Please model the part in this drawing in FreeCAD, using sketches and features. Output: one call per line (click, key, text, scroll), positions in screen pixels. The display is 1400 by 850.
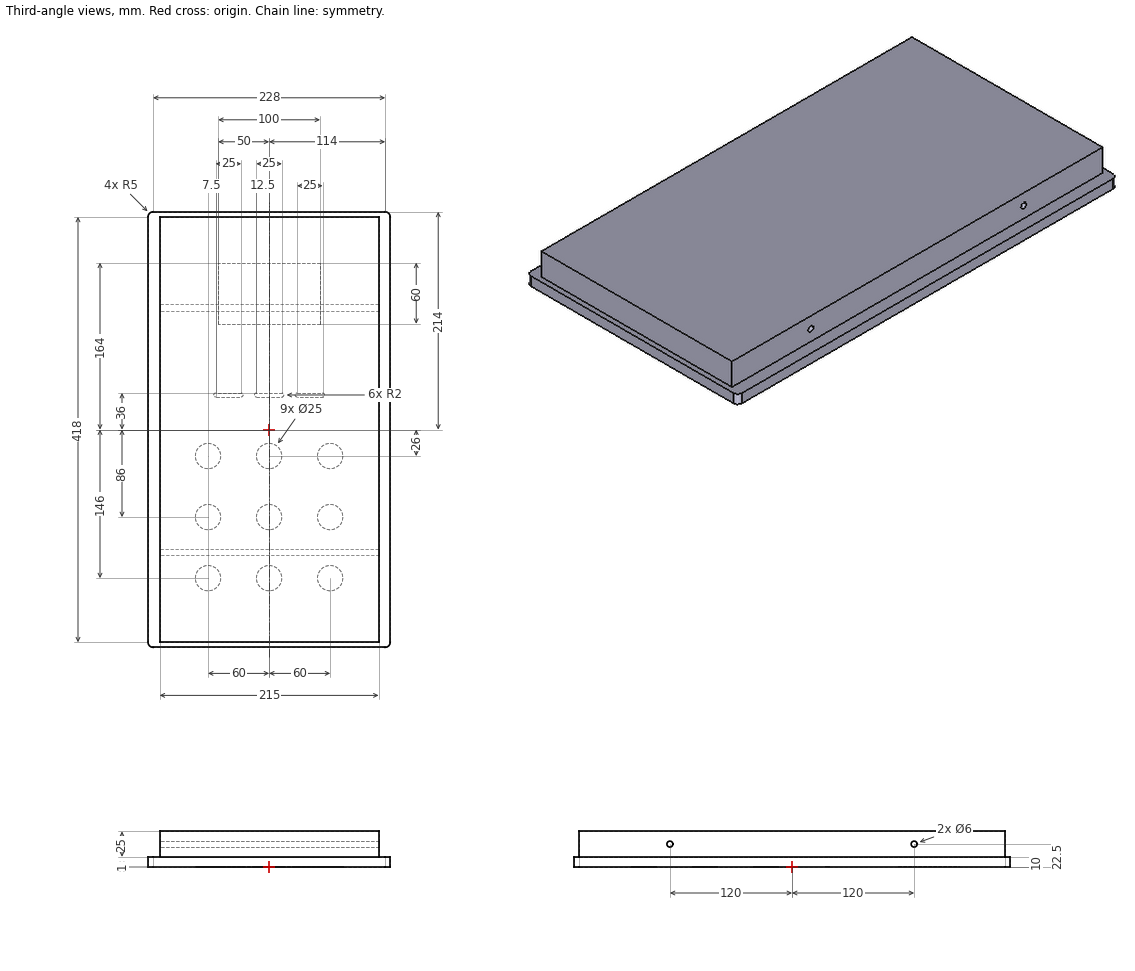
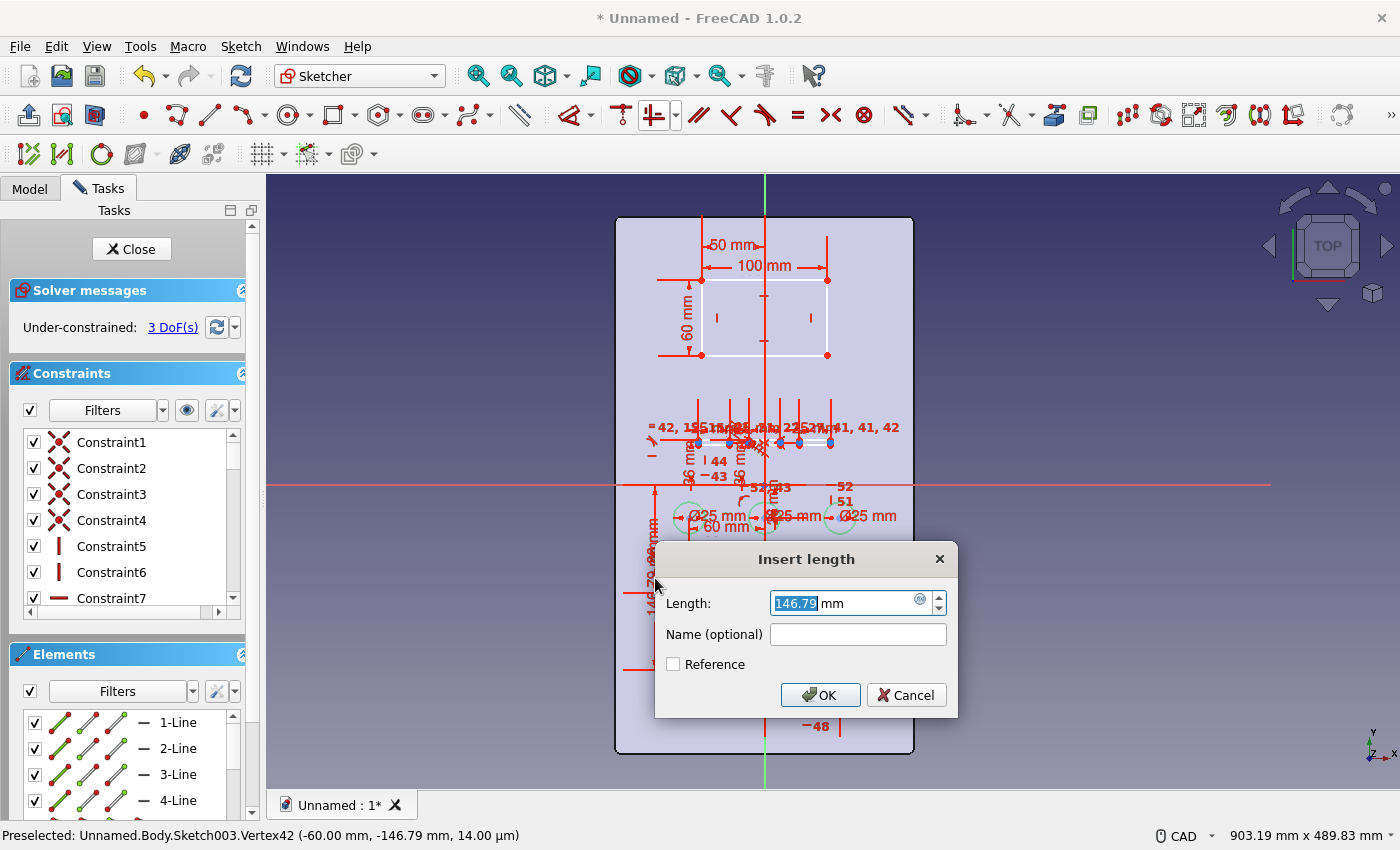
text(146)
key(Return)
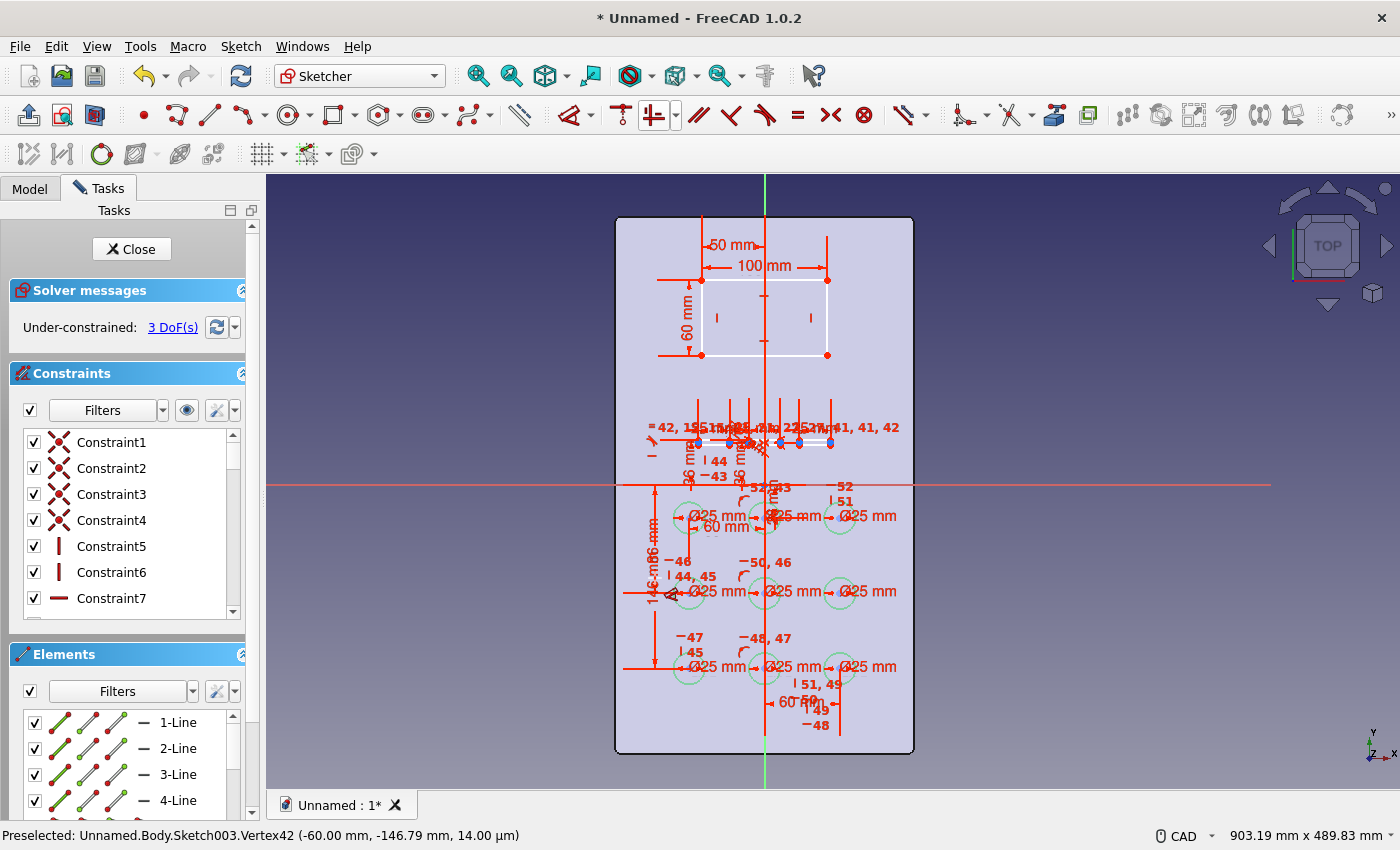
click(702, 280)
click(668, 383)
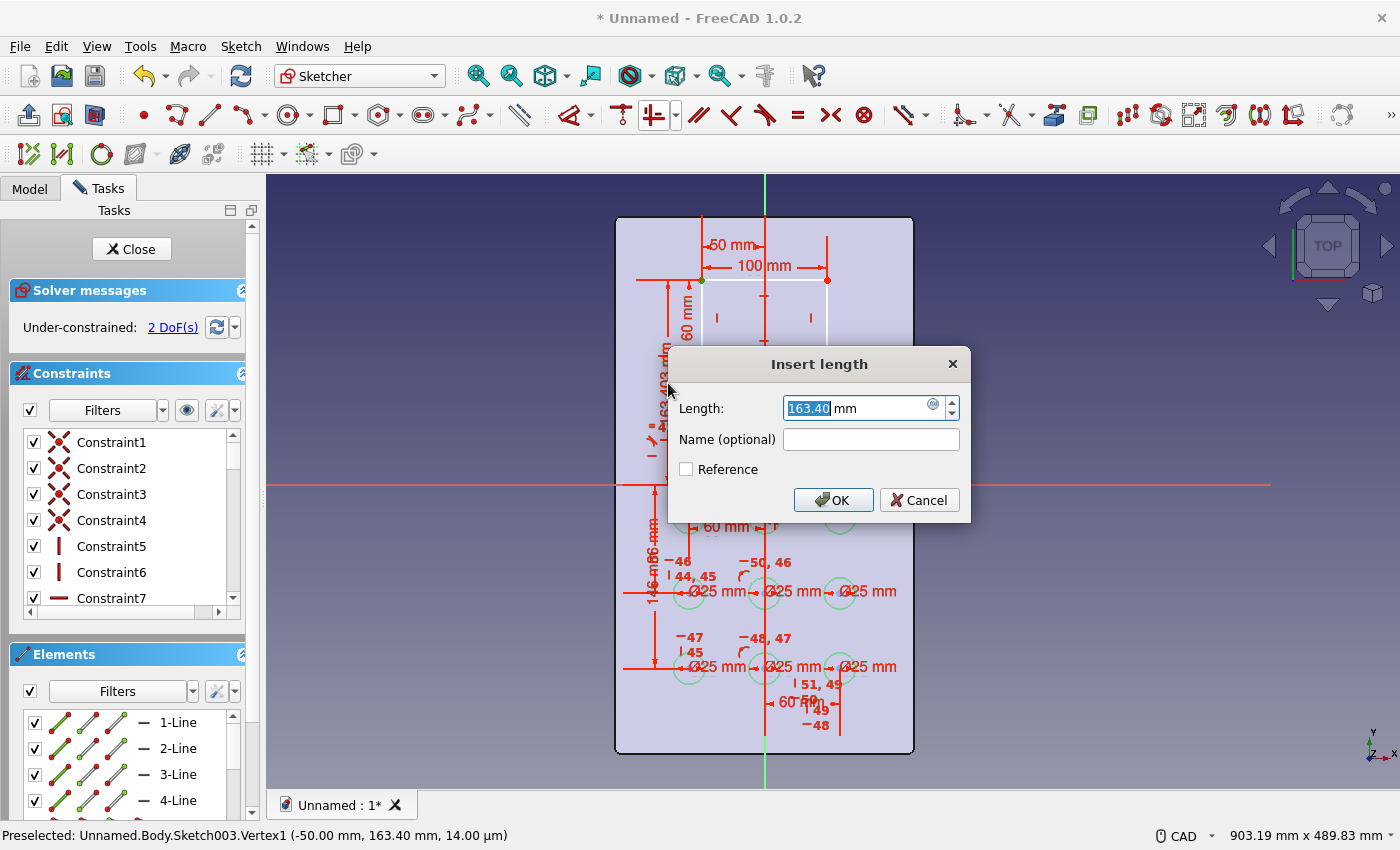
text(164)
key(Return)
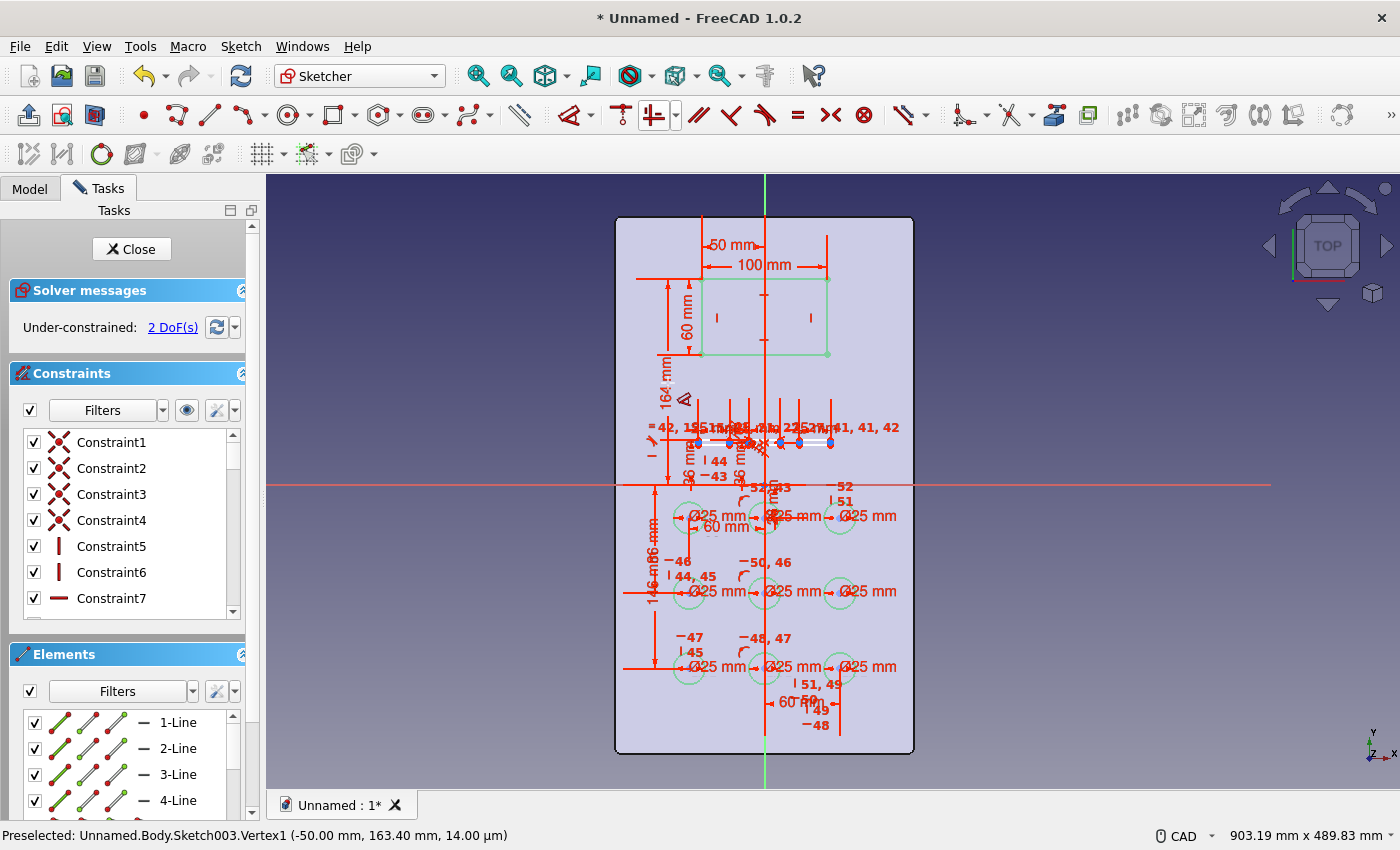
scroll(698, 445, up, 8)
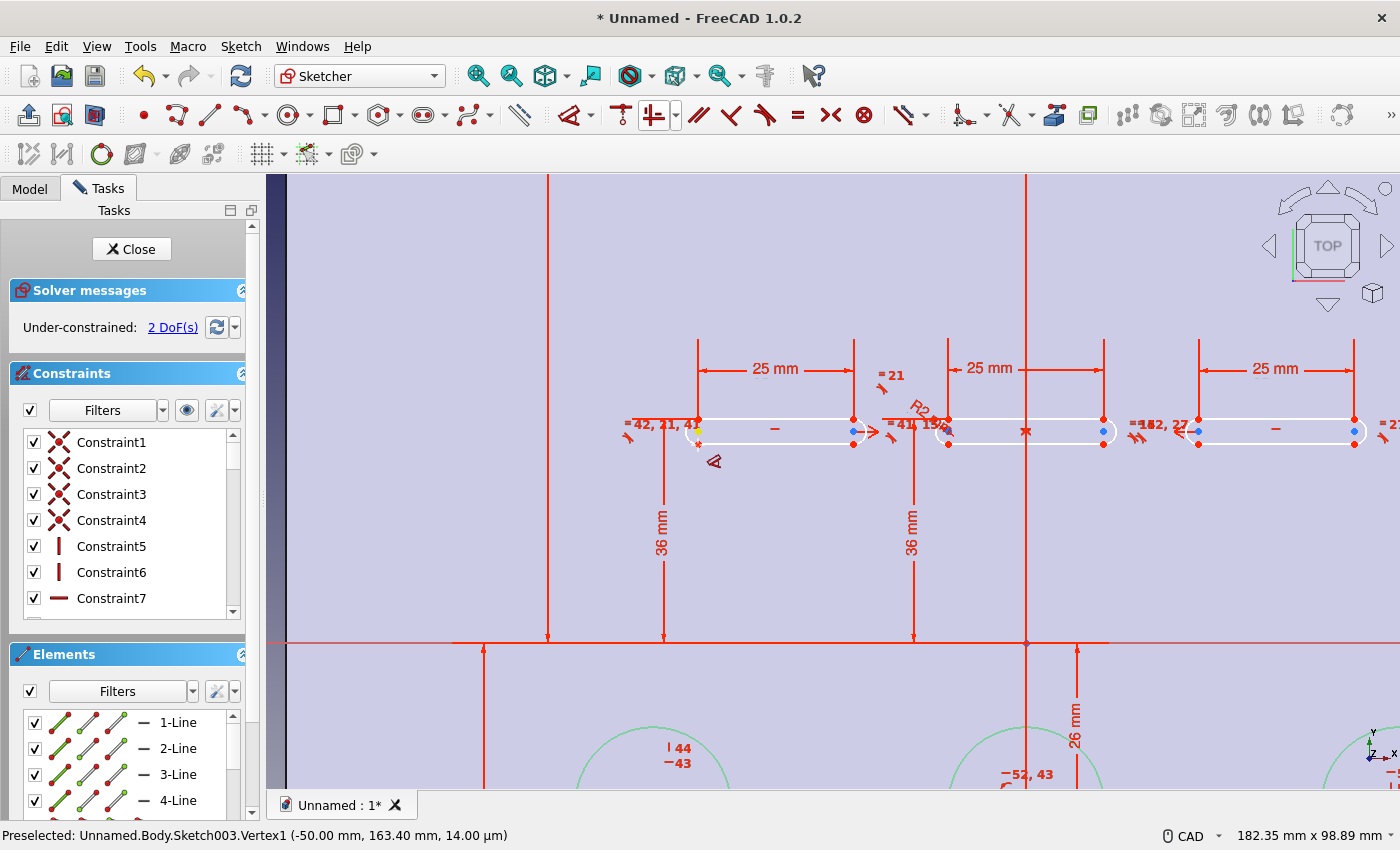
click(698, 444)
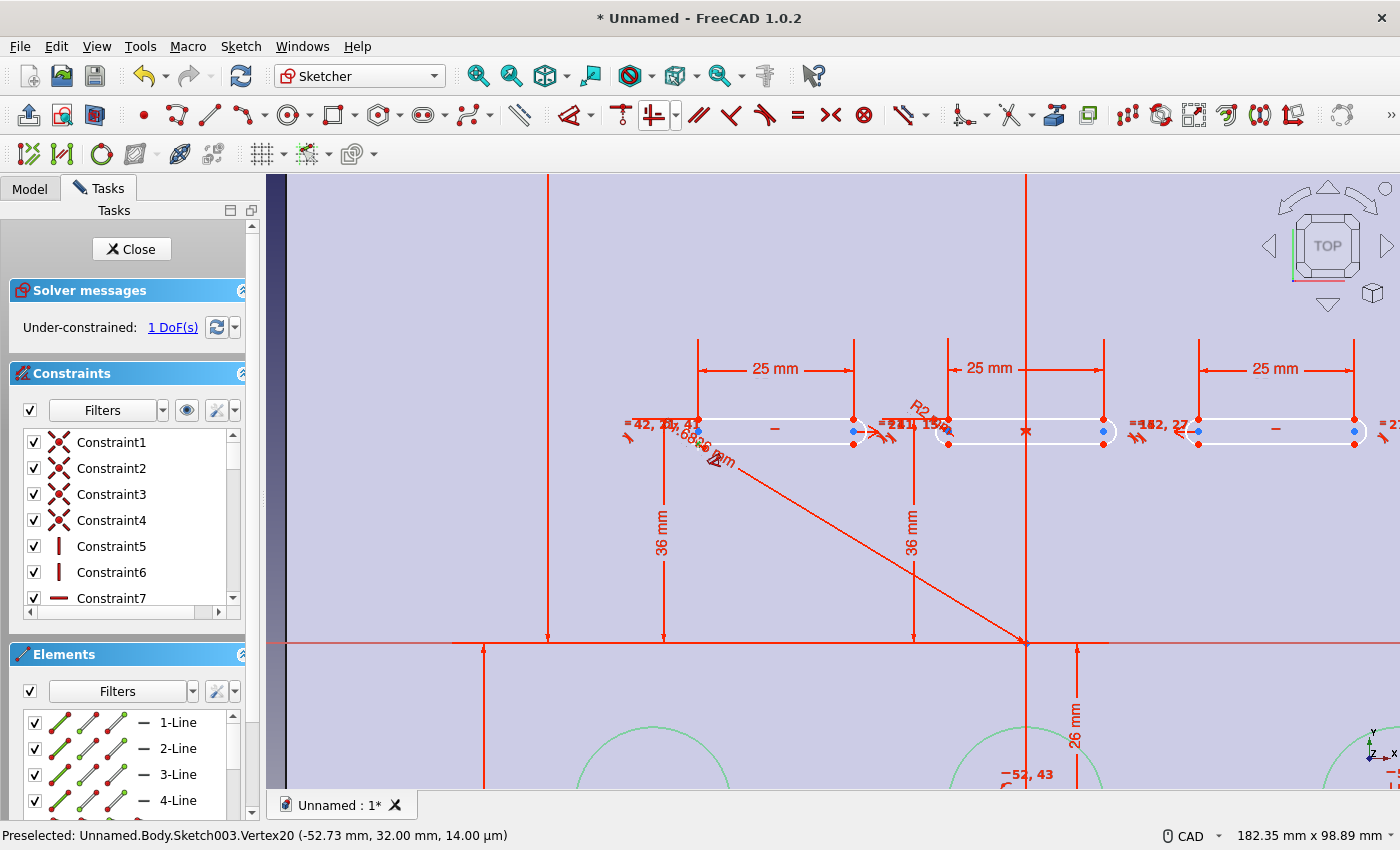
scroll(698, 445, down, 8)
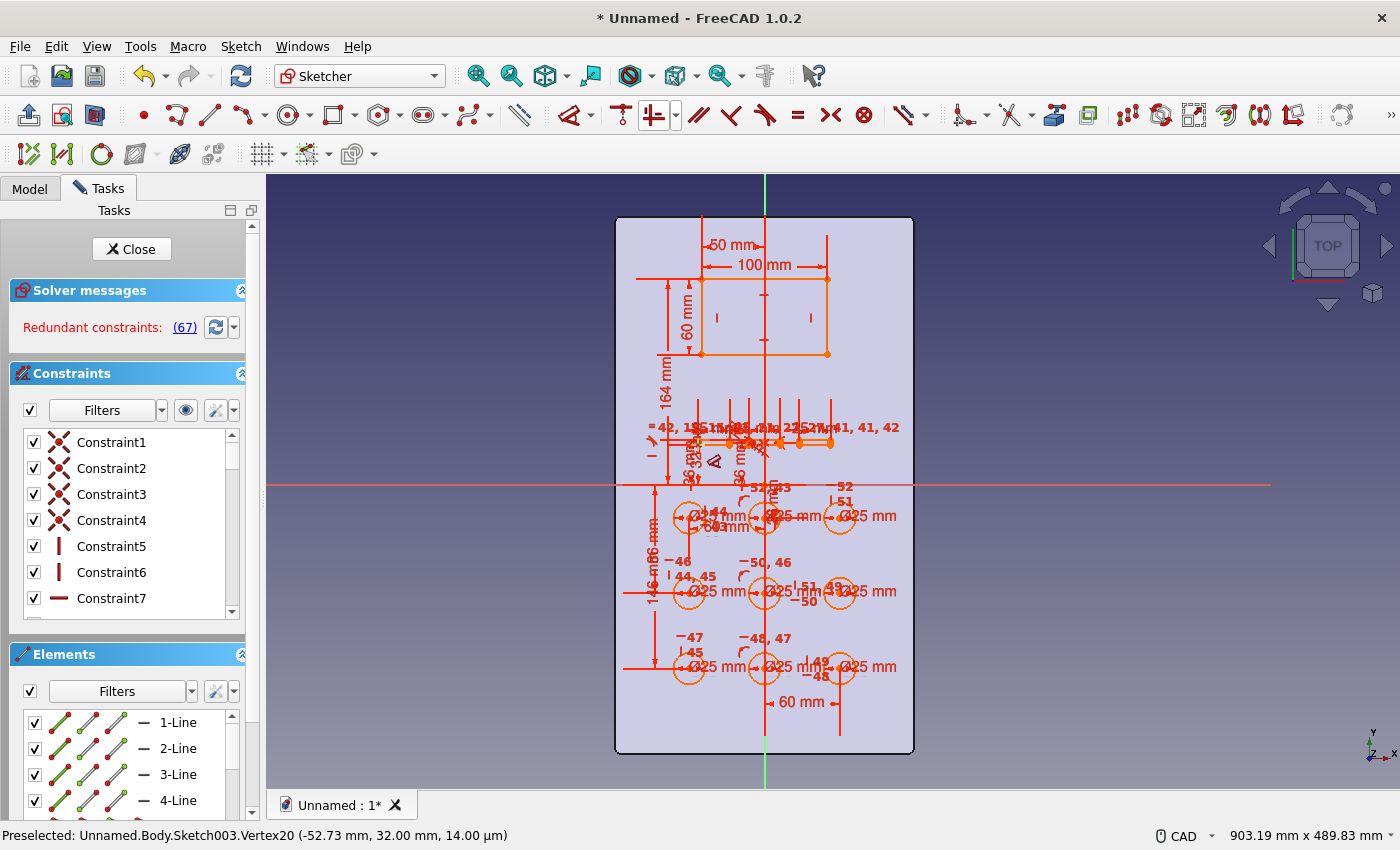
scroll(689, 518, up, 8)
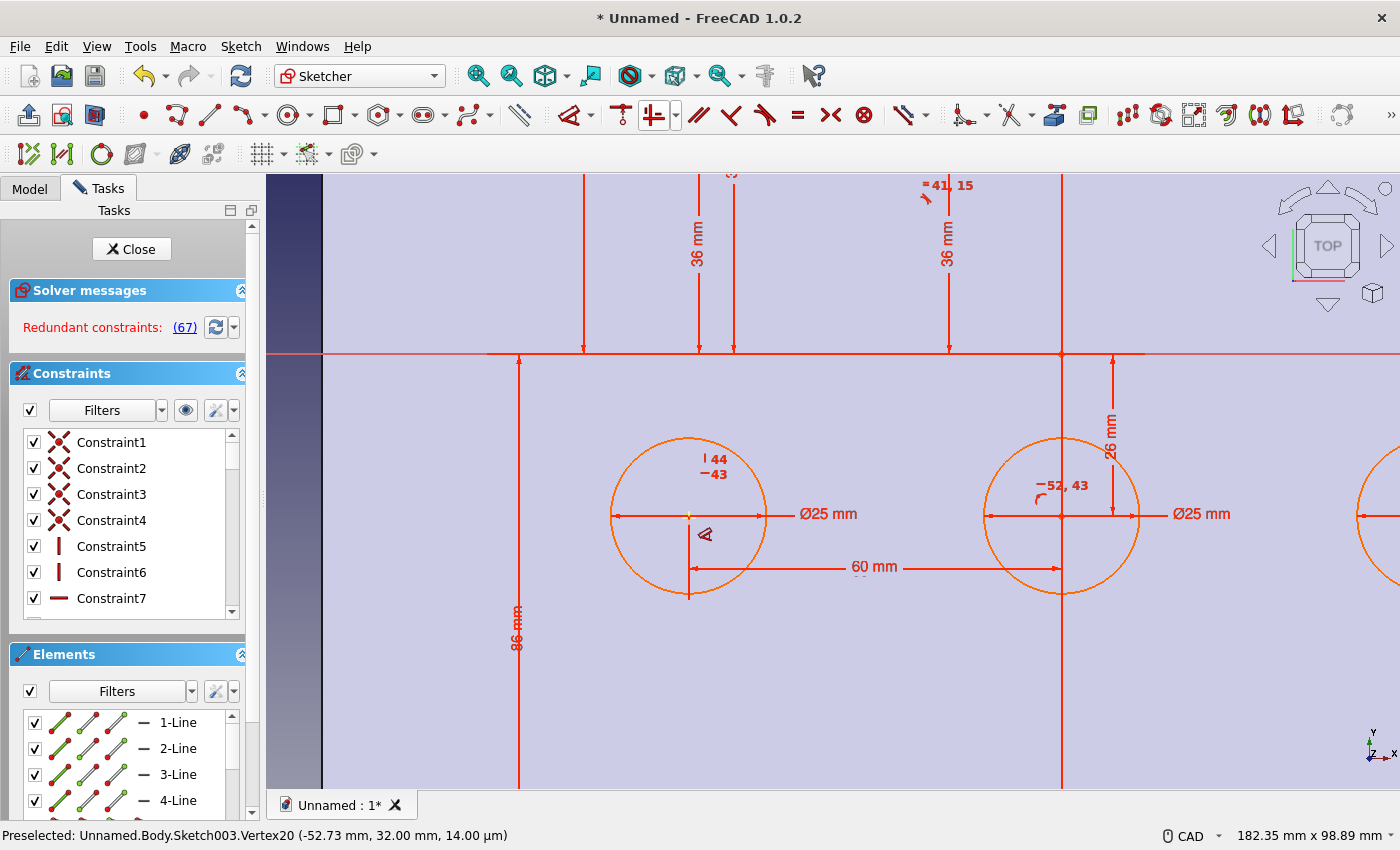
click(689, 516)
click(711, 550)